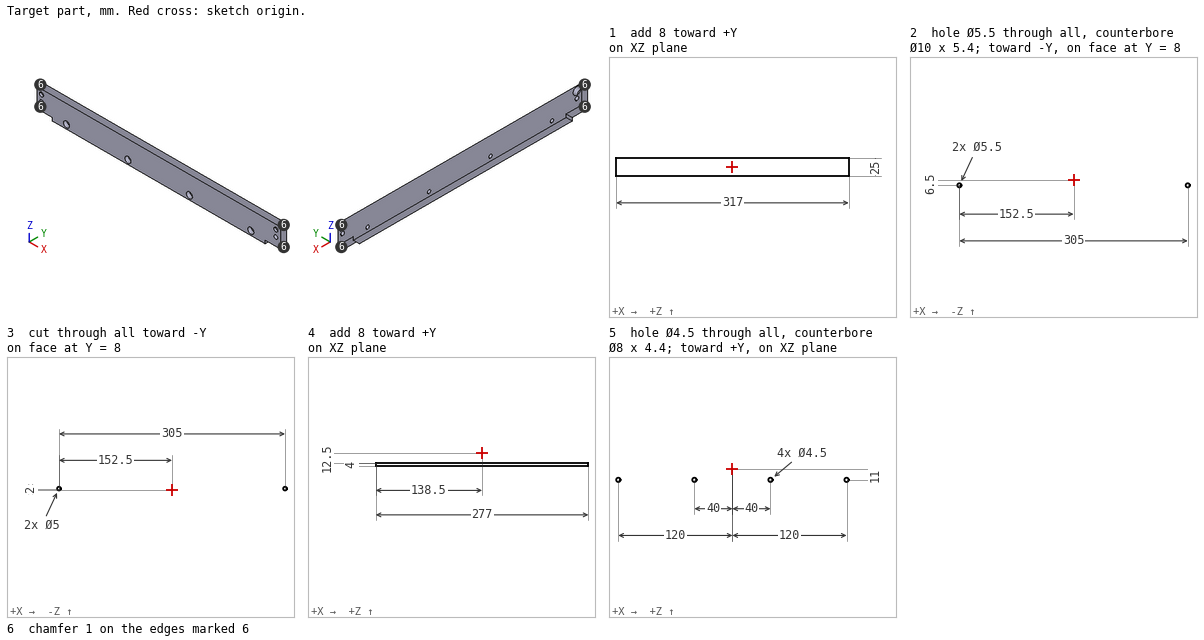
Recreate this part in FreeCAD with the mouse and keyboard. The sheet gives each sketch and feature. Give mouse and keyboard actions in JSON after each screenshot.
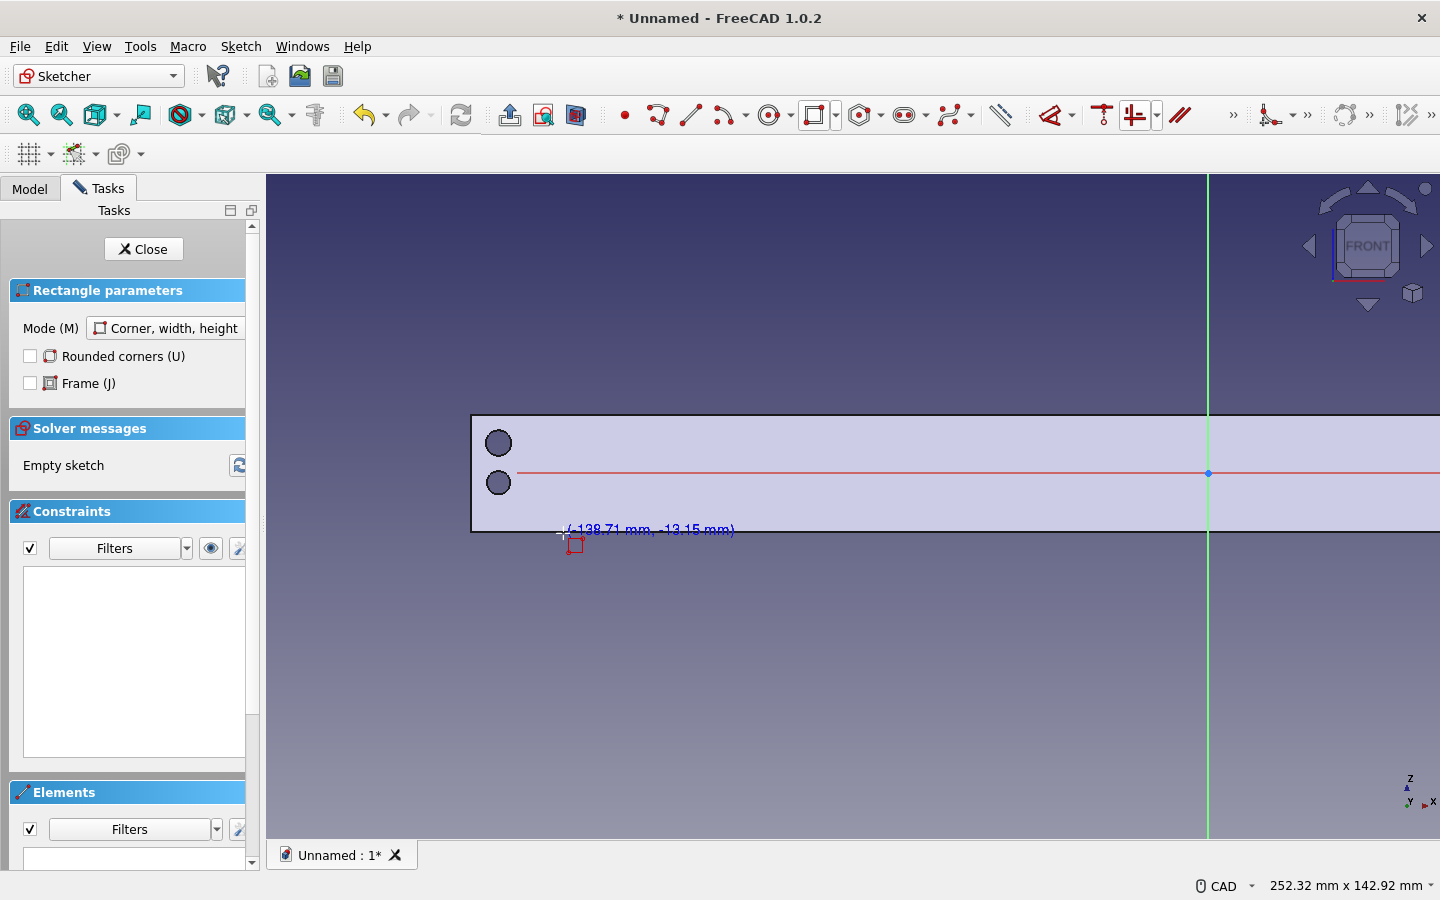
{"action": "left_click", "coordinate": [564, 532]}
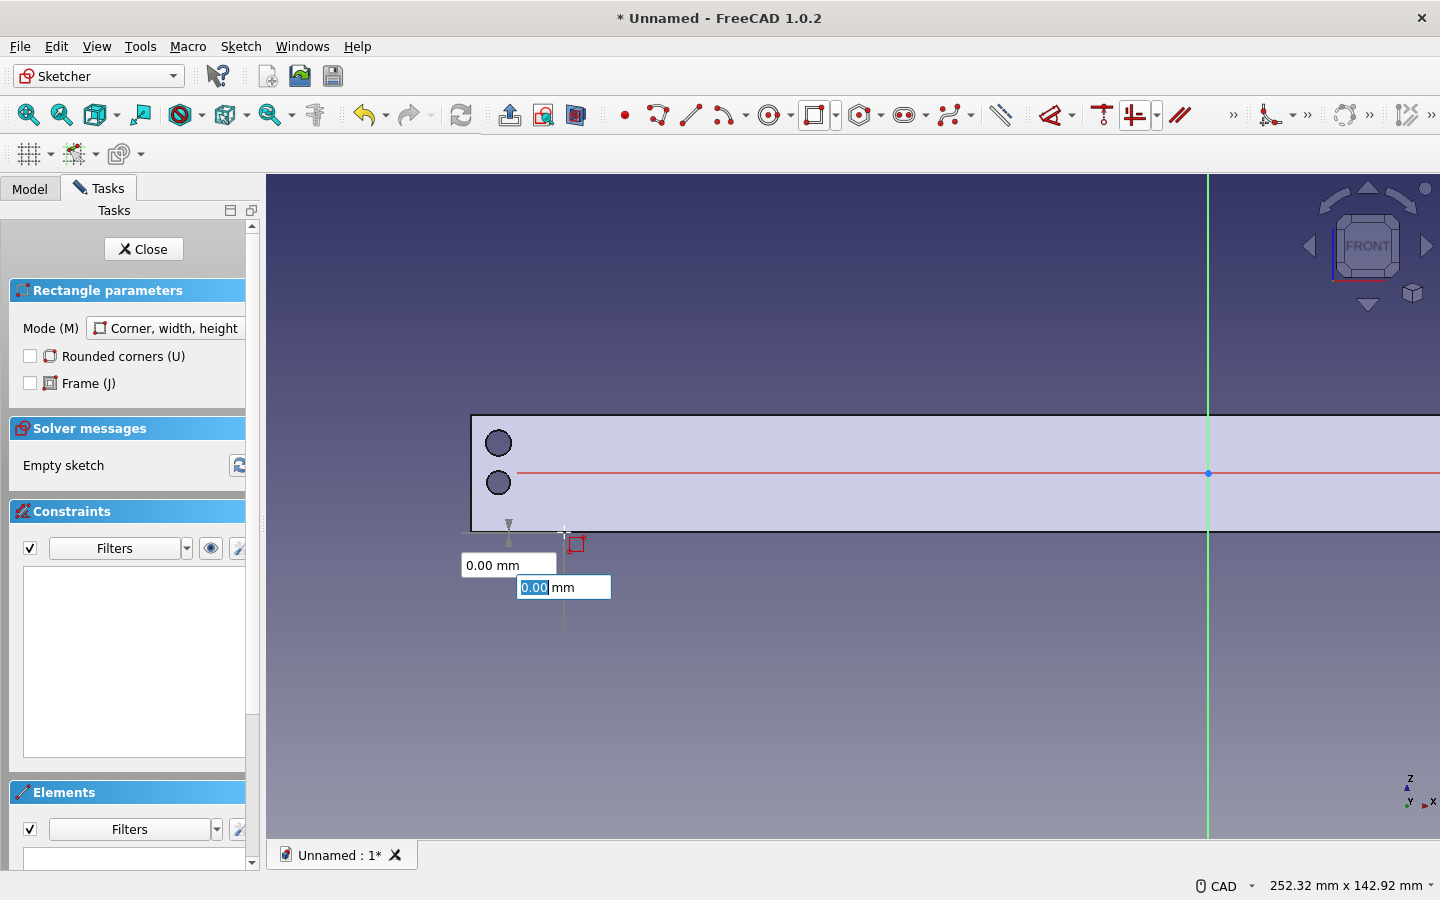
{"action": "scroll", "coordinate": [294, 500], "scroll_direction": "down", "scroll_amount": 3}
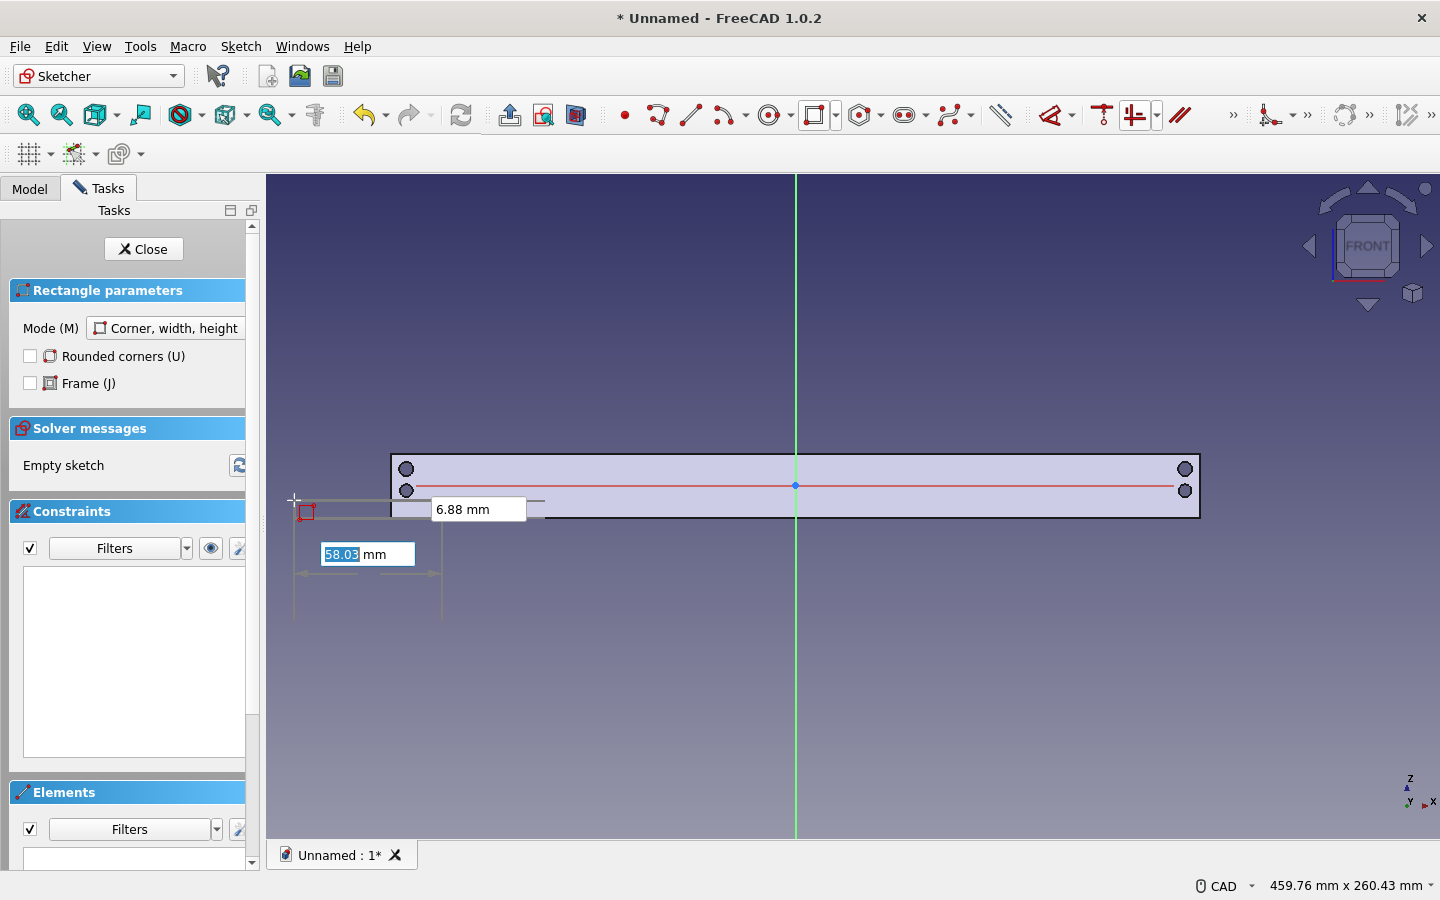
{"action": "left_click", "coordinate": [1149, 528]}
{"action": "key", "text": "Escape"}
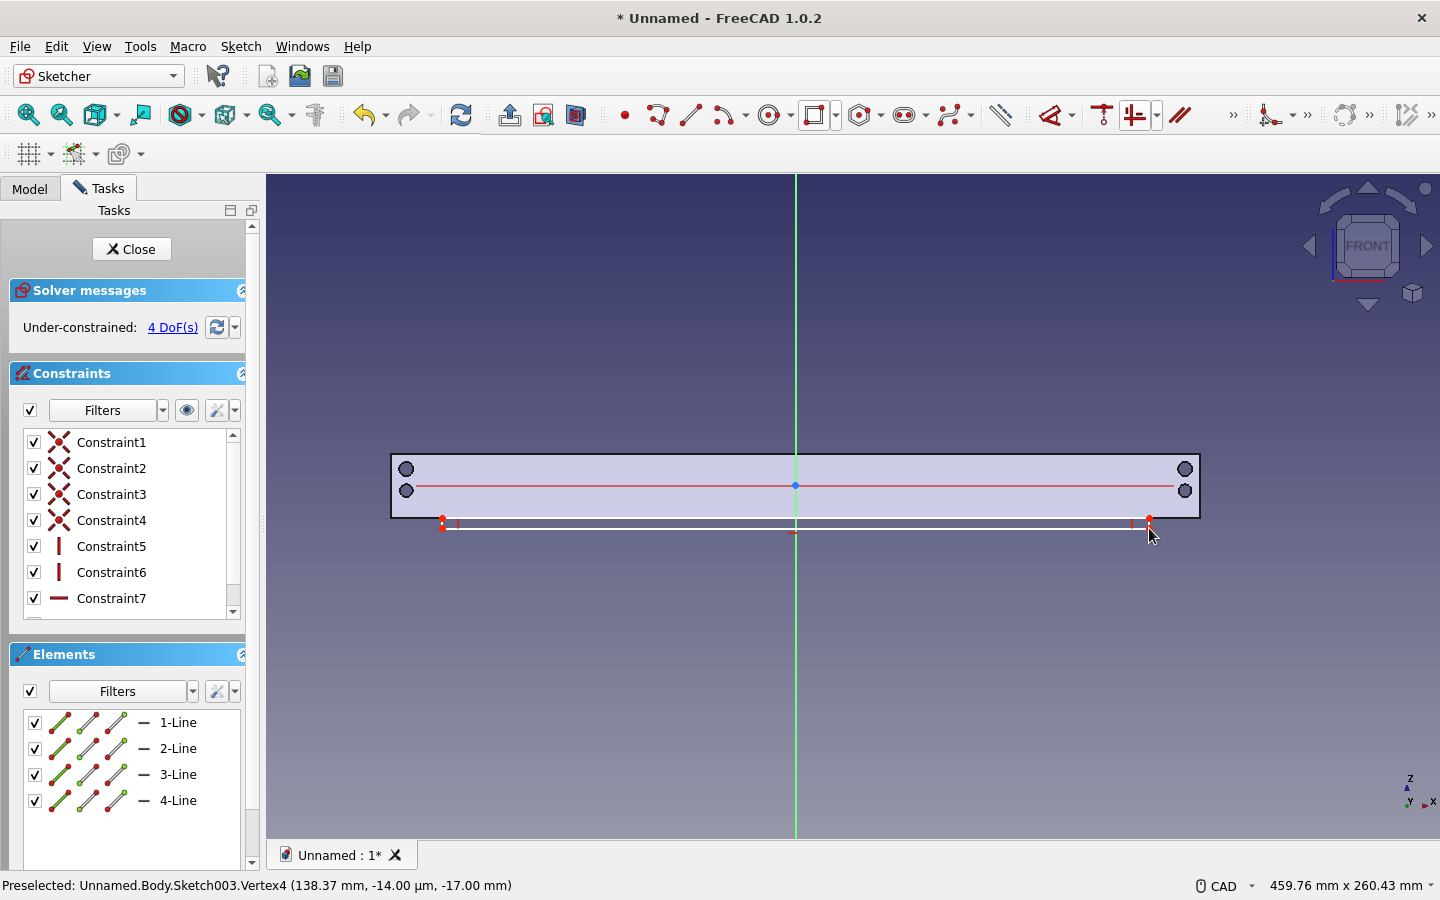
{"action": "left_click", "coordinate": [1050, 116]}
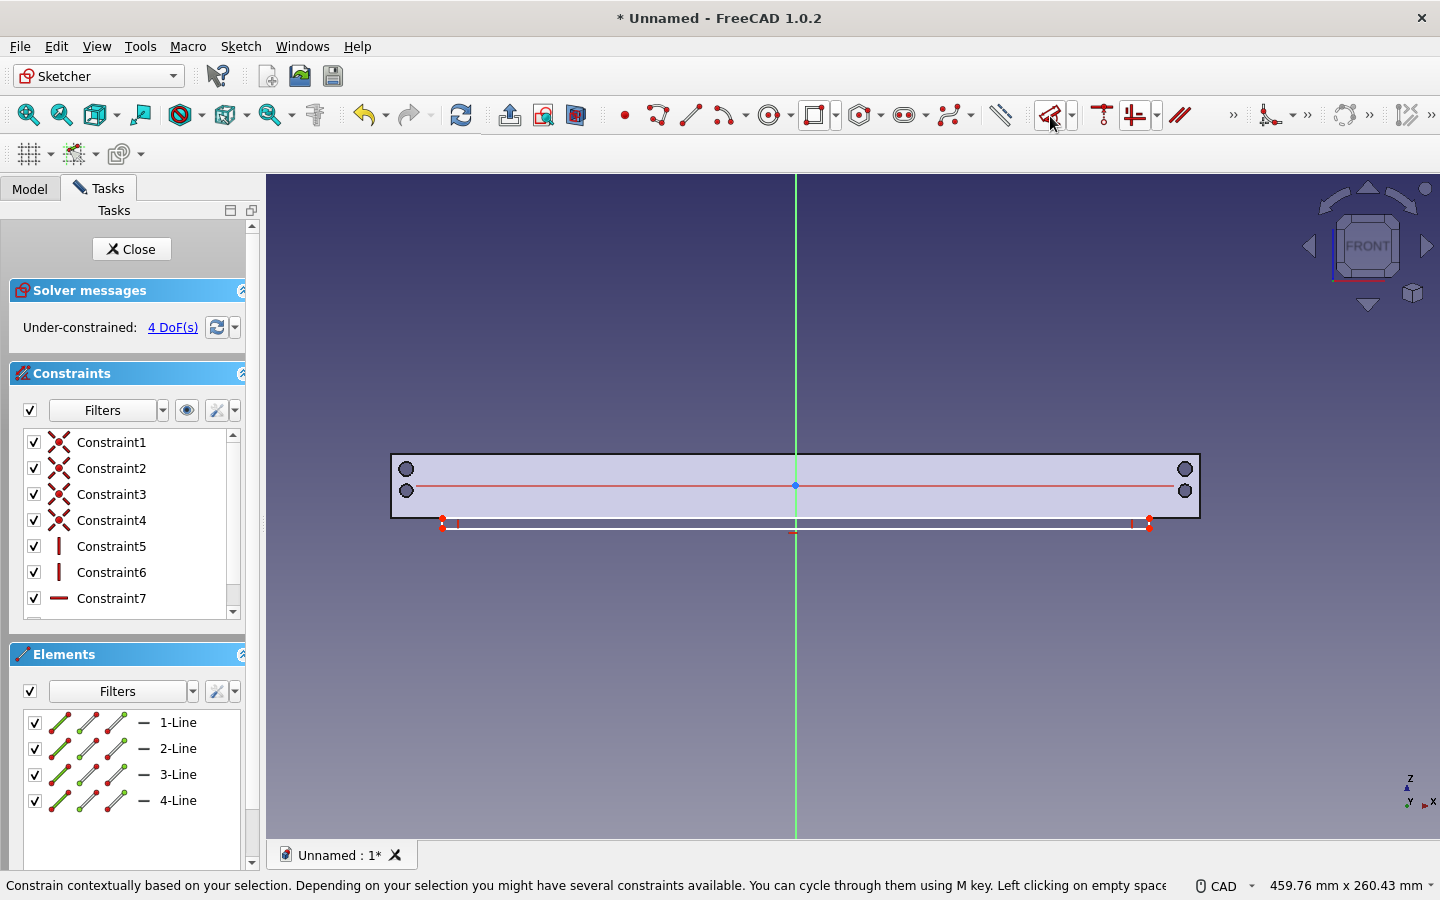
{"action": "scroll", "coordinate": [442, 524], "scroll_direction": "up", "scroll_amount": 7}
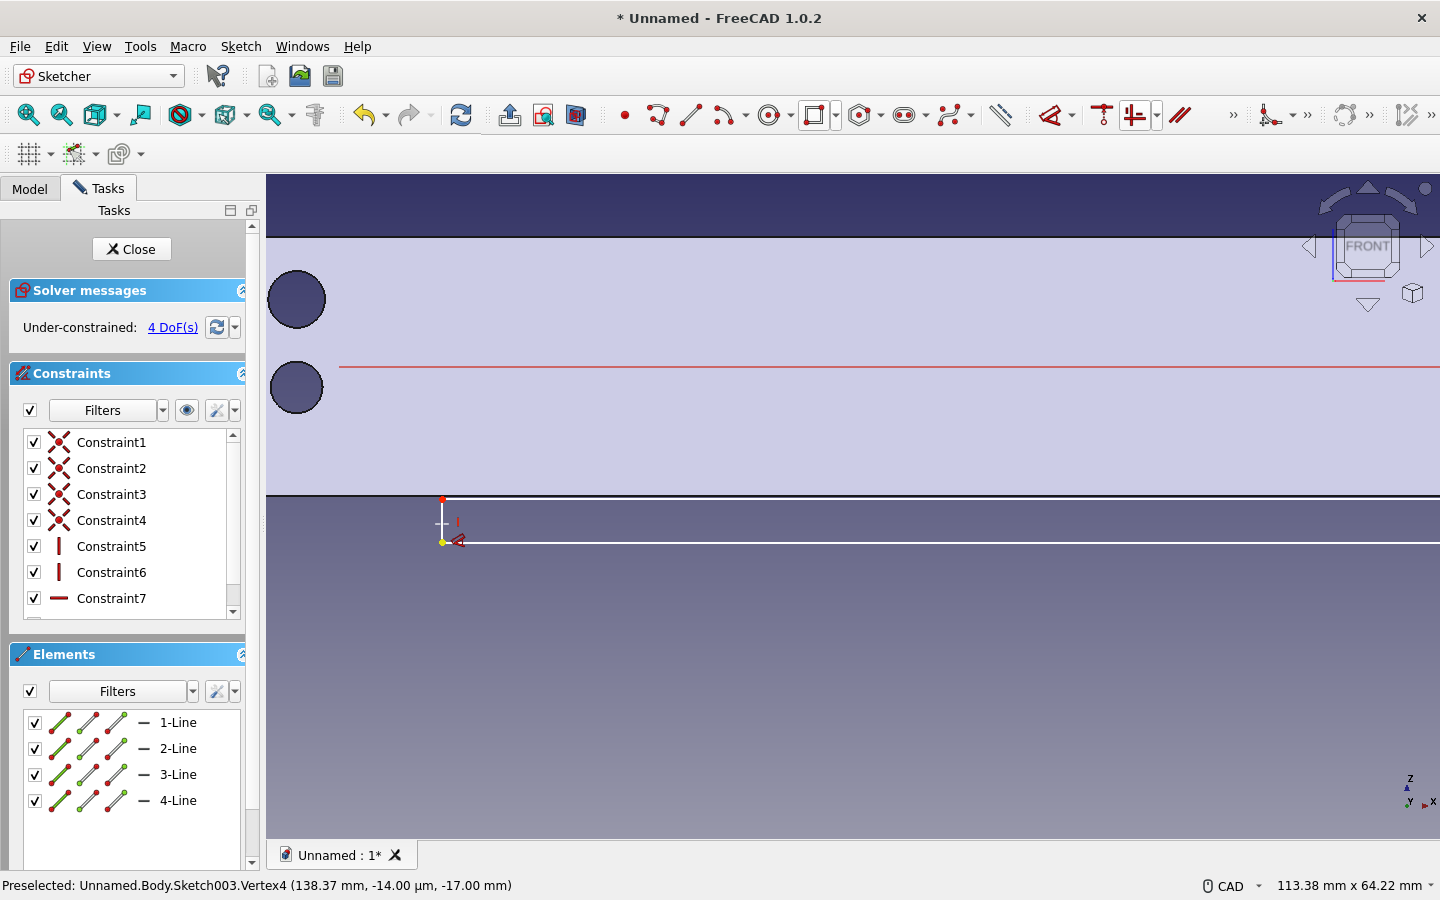
{"action": "left_click", "coordinate": [442, 521]}
{"action": "left_click", "coordinate": [408, 521]}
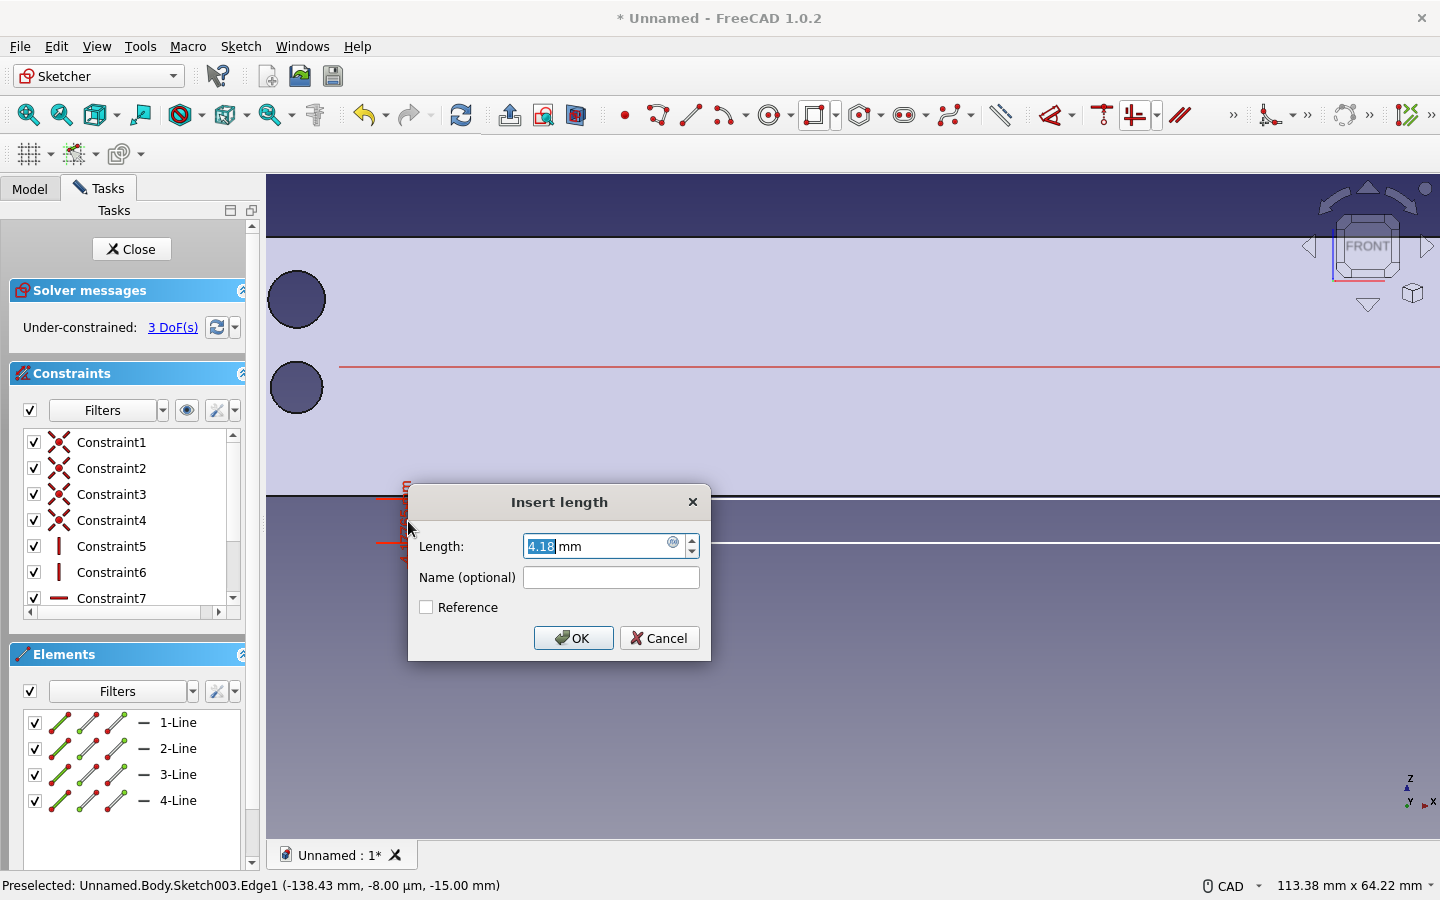
{"action": "type", "text": "4"}
{"action": "key", "text": "Return"}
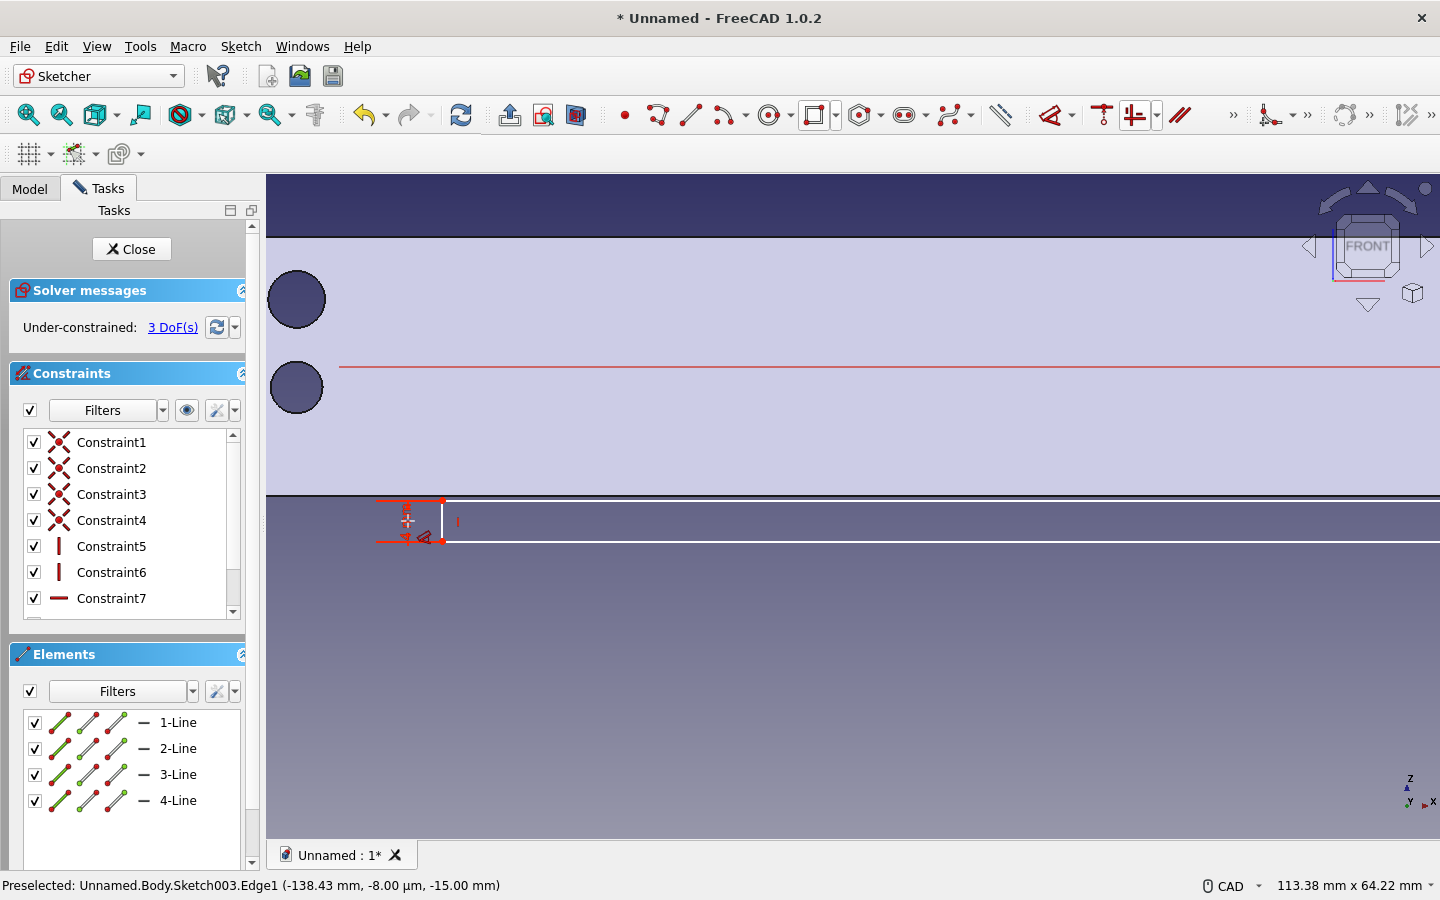
{"action": "scroll", "coordinate": [427, 524], "scroll_direction": "down", "scroll_amount": 7}